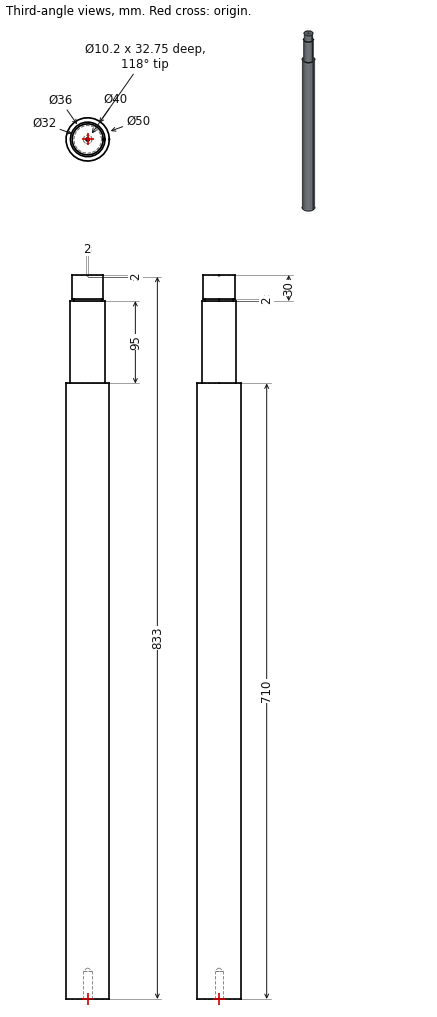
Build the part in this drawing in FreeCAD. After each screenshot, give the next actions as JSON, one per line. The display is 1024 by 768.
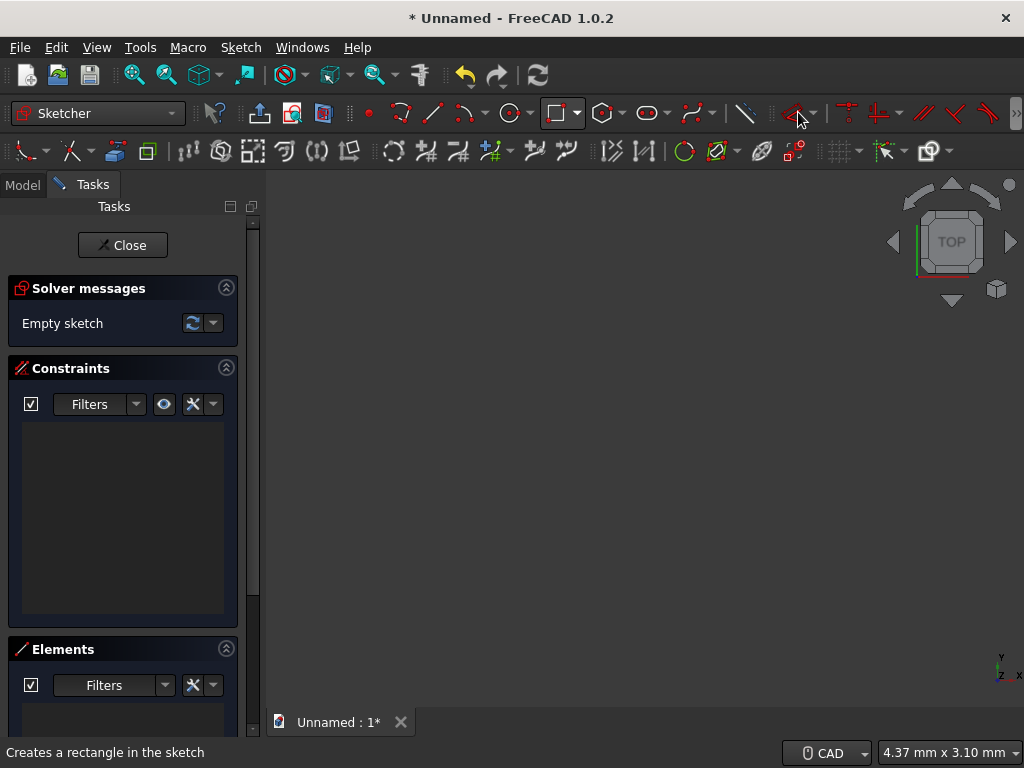
{"action": "scroll", "coordinate": [576, 438], "scroll_direction": "down", "scroll_amount": 15}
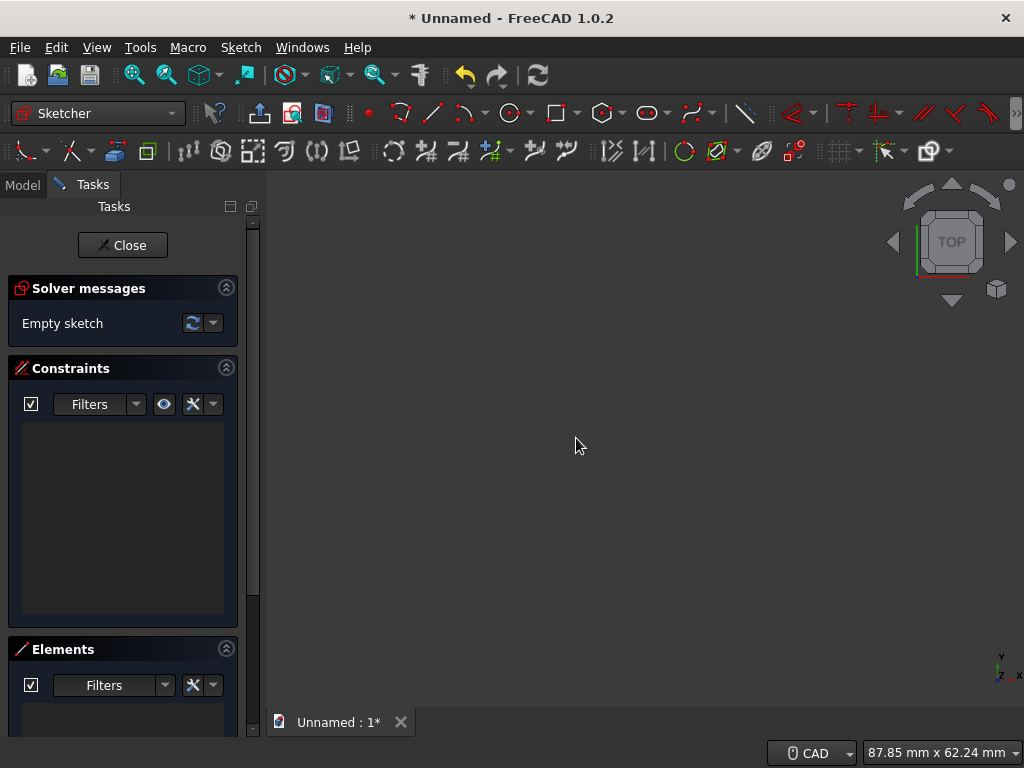
{"action": "scroll", "coordinate": [576, 438], "scroll_direction": "down", "scroll_amount": 5}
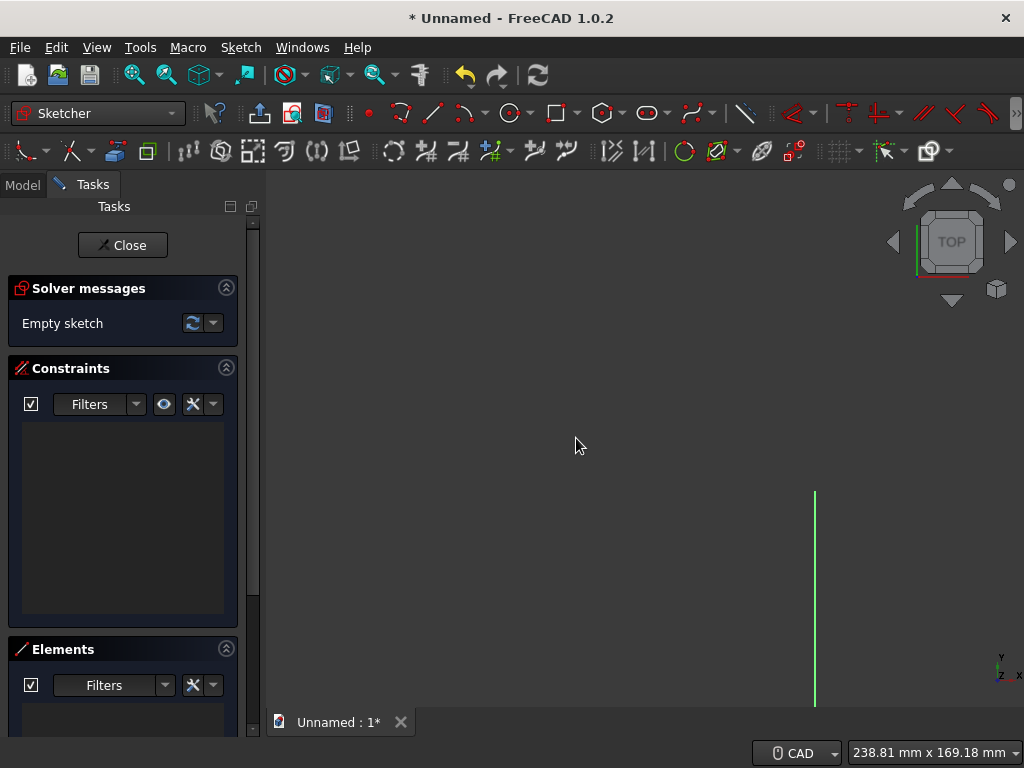
{"action": "scroll", "coordinate": [576, 438], "scroll_direction": "down", "scroll_amount": 5}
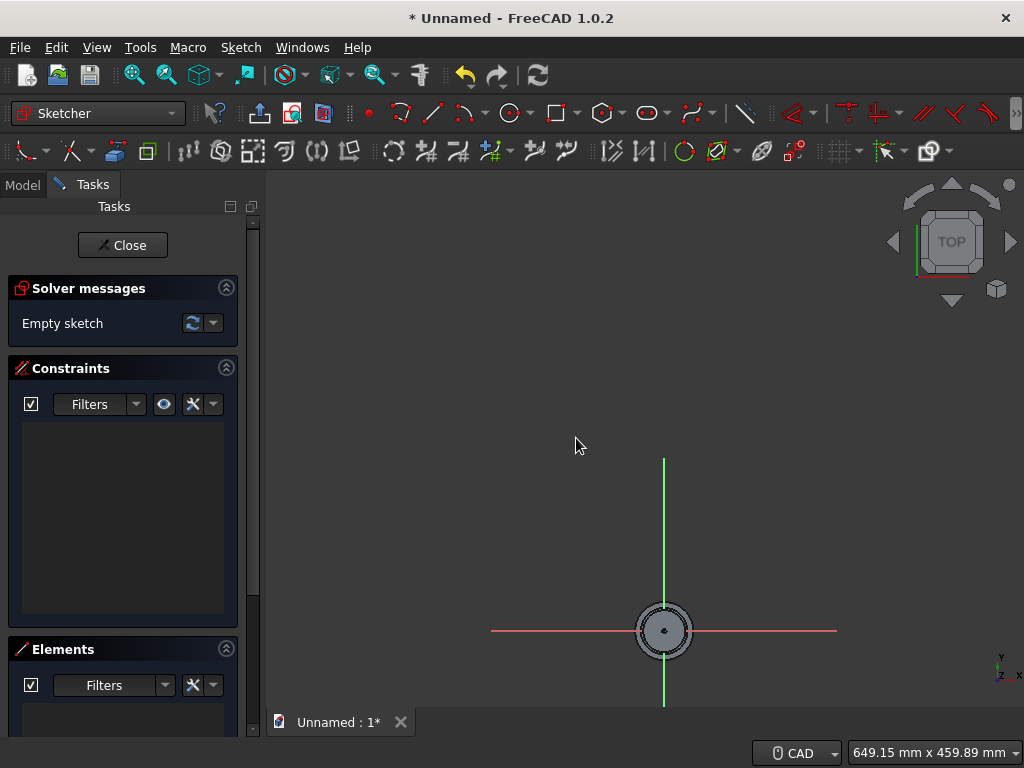
{"action": "scroll", "coordinate": [678, 661], "scroll_direction": "up", "scroll_amount": 10}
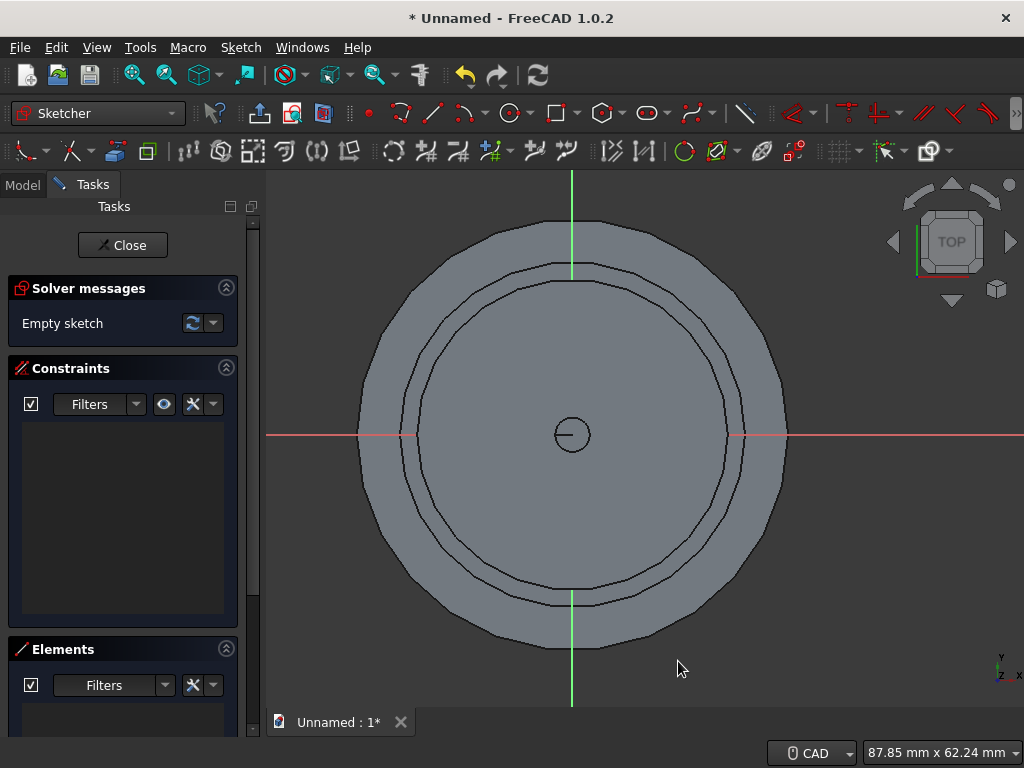
{"action": "left_click", "coordinate": [510, 114]}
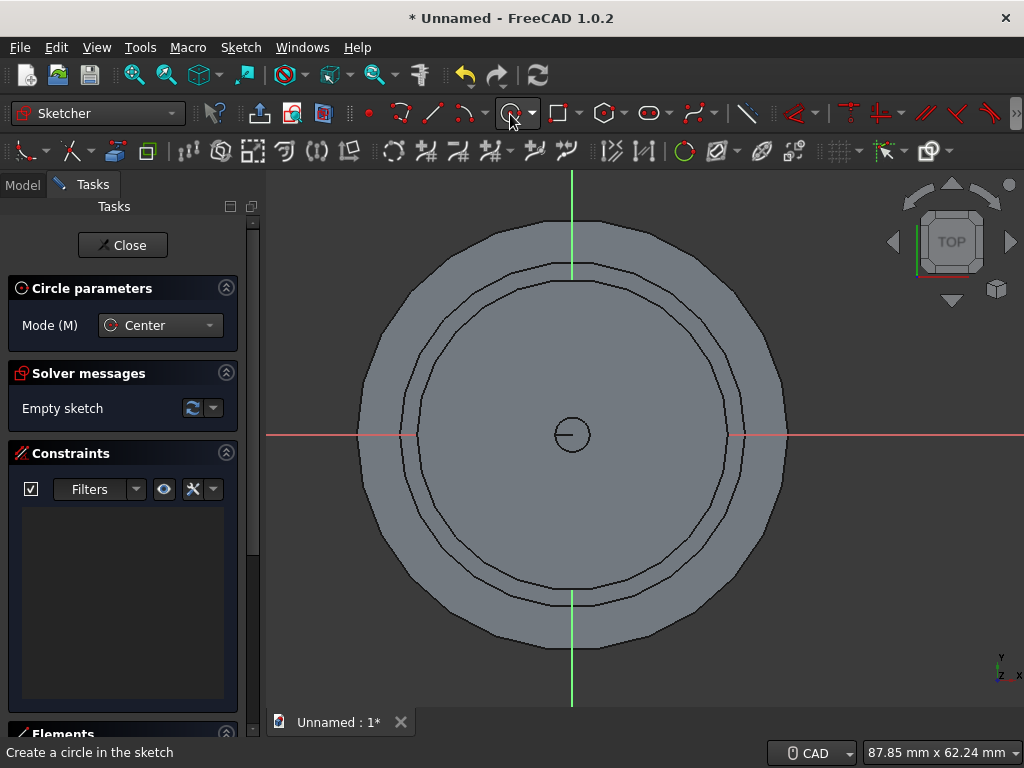
{"action": "left_click", "coordinate": [572, 435]}
{"action": "mouse_move", "coordinate": [695, 313]}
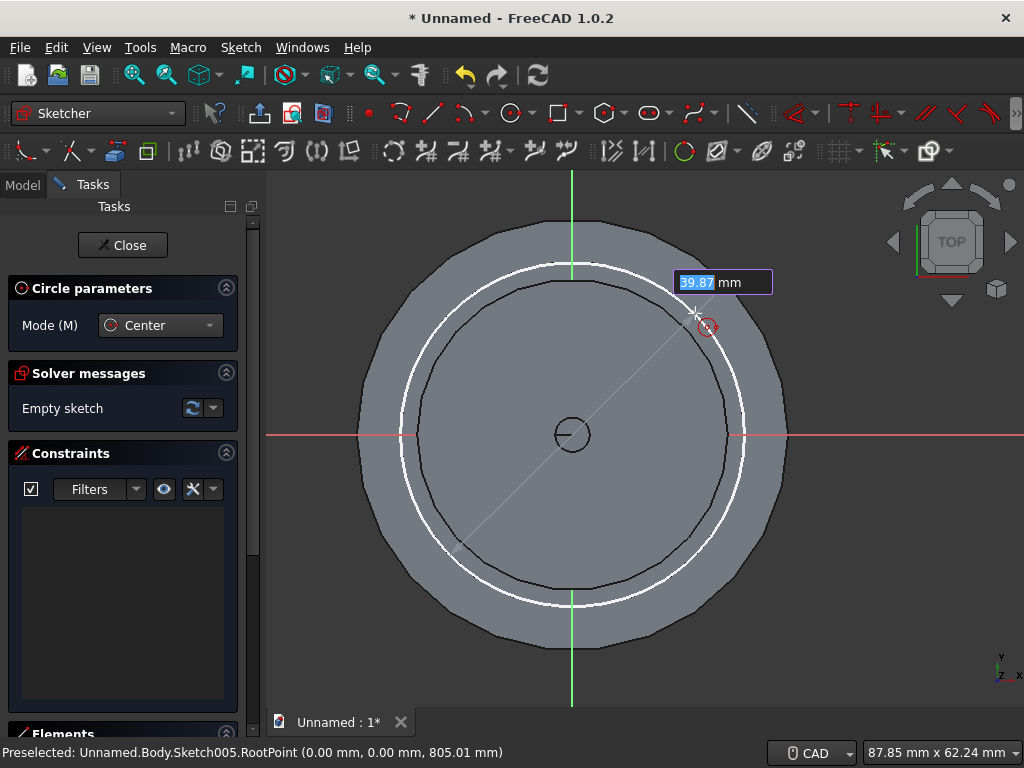
{"action": "type", "text": "40"}
{"action": "key", "text": "Return"}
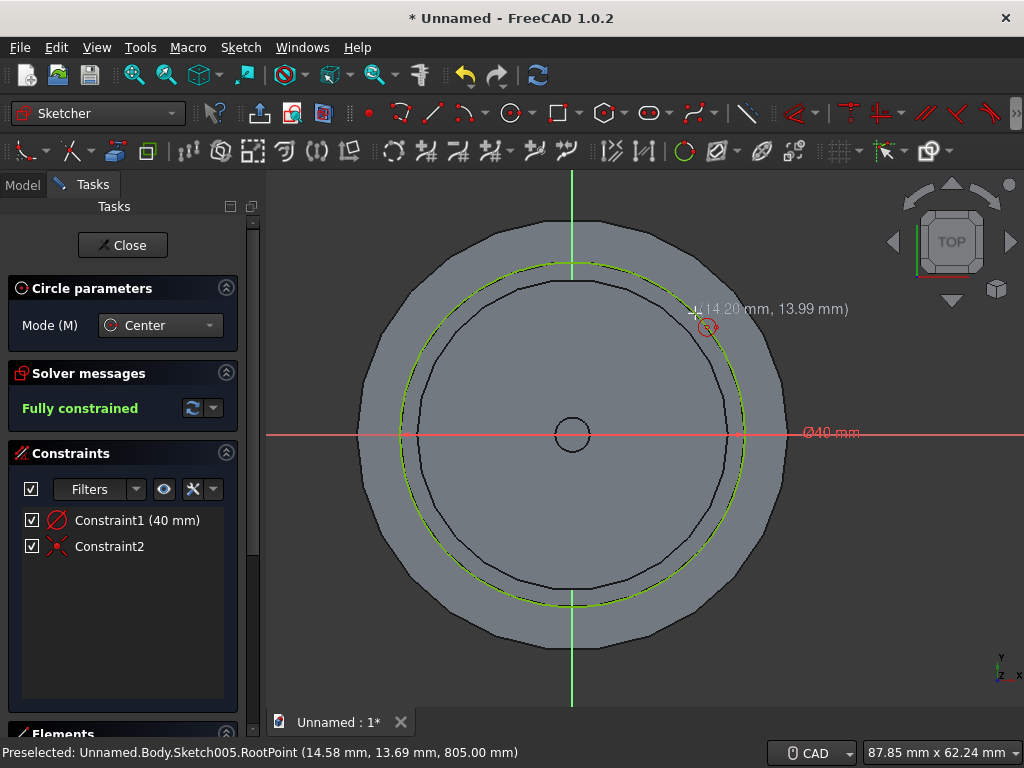
{"action": "left_click", "coordinate": [572, 435]}
{"action": "mouse_move", "coordinate": [670, 337]}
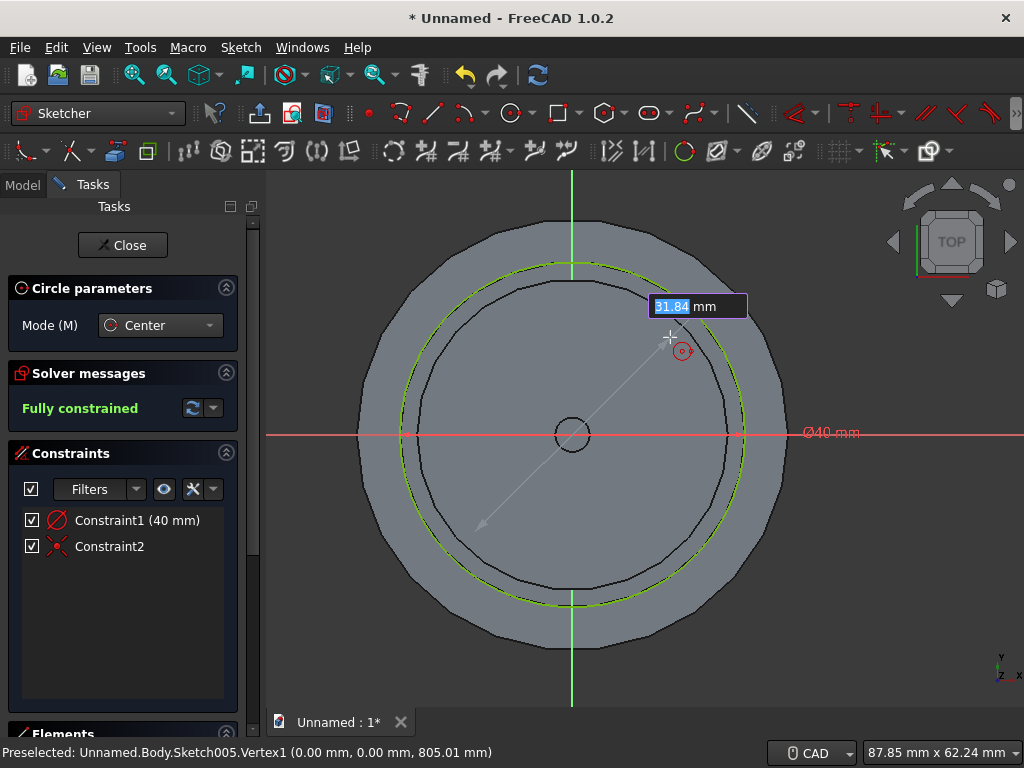
{"action": "type", "text": "32"}
{"action": "key", "text": "Return"}
{"action": "key", "text": "Escape"}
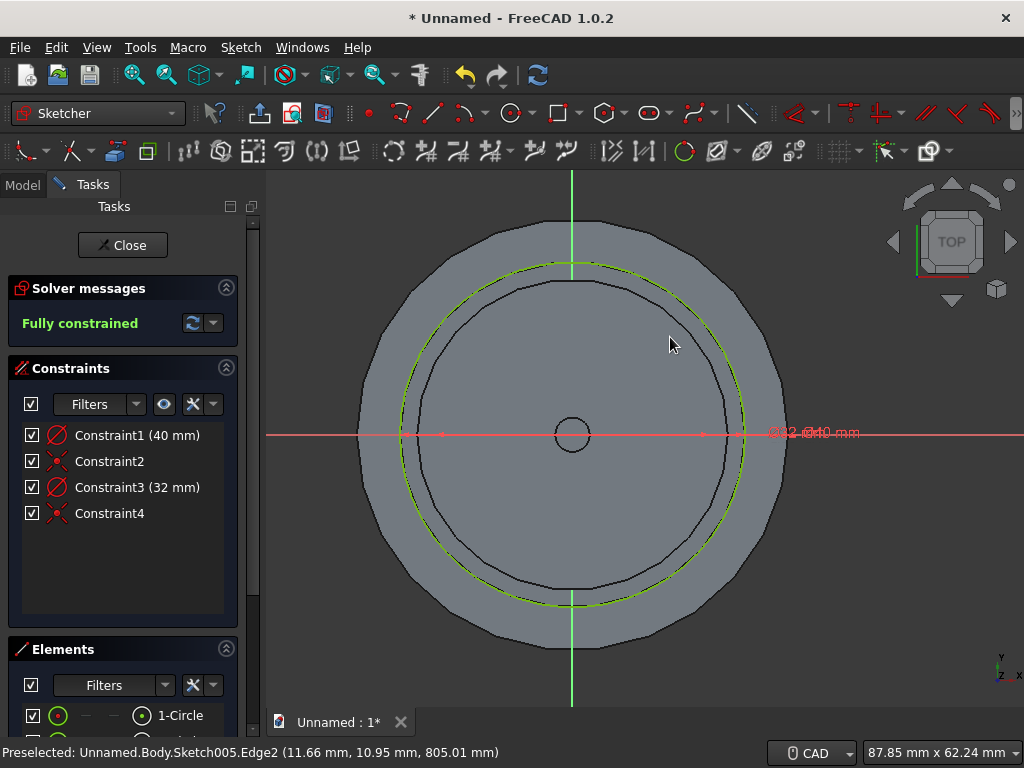
{"action": "left_click", "coordinate": [123, 245]}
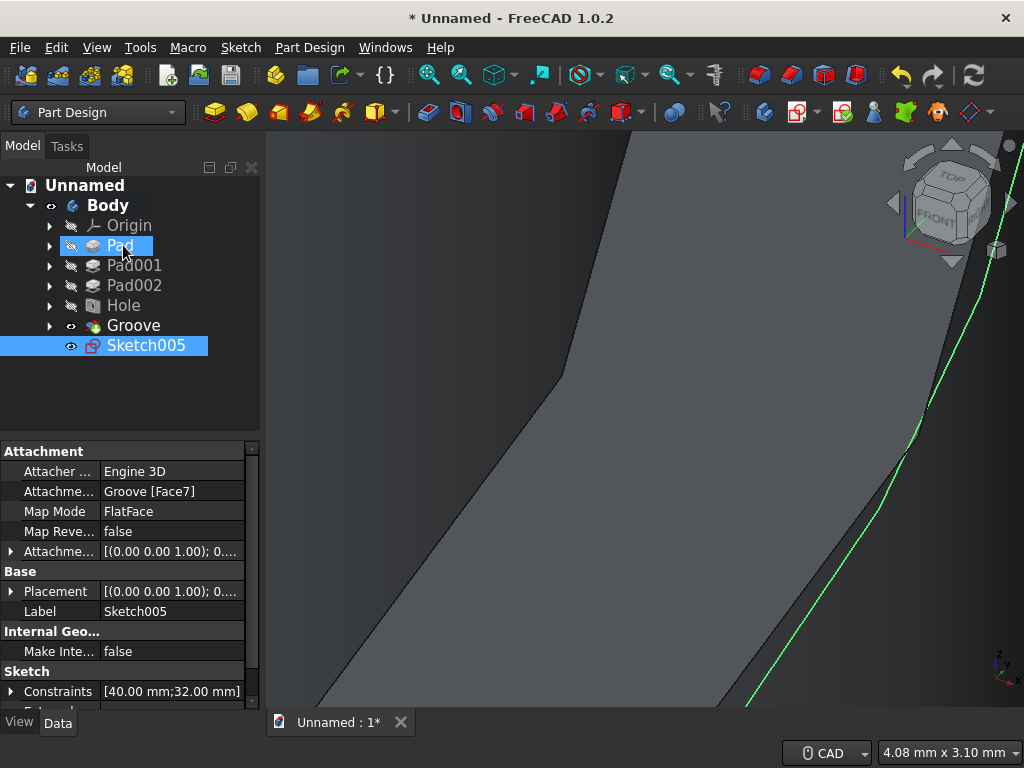
{"action": "left_click", "coordinate": [430, 112]}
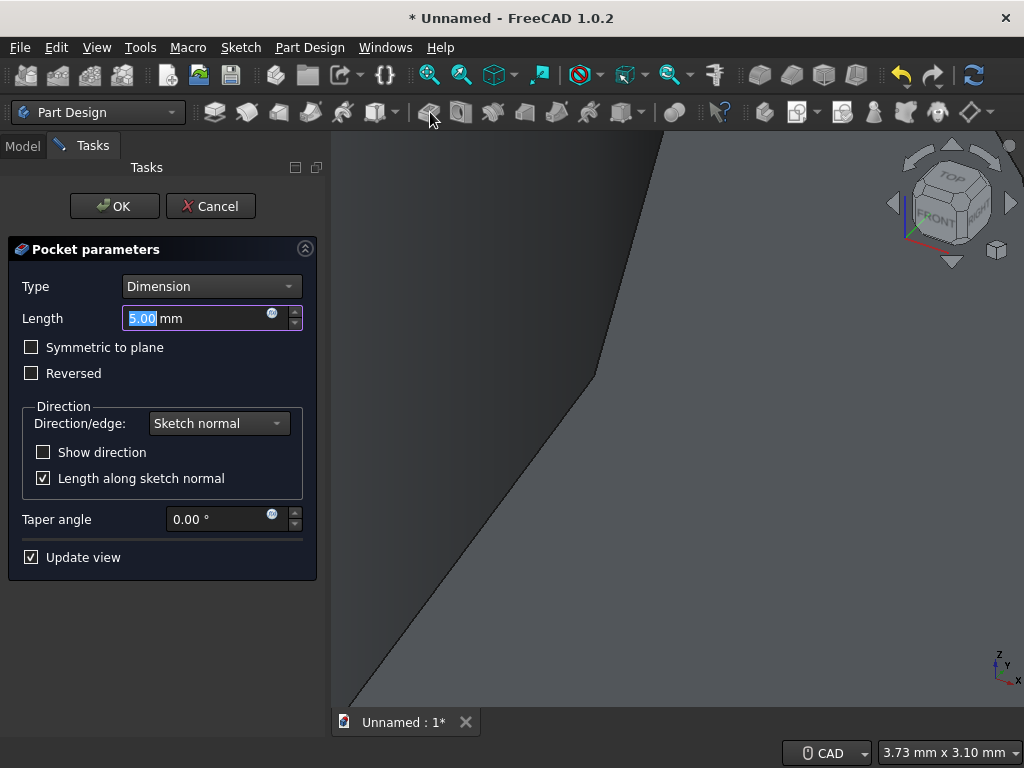
{"action": "type", "text": "2"}
{"action": "key", "text": "Tab"}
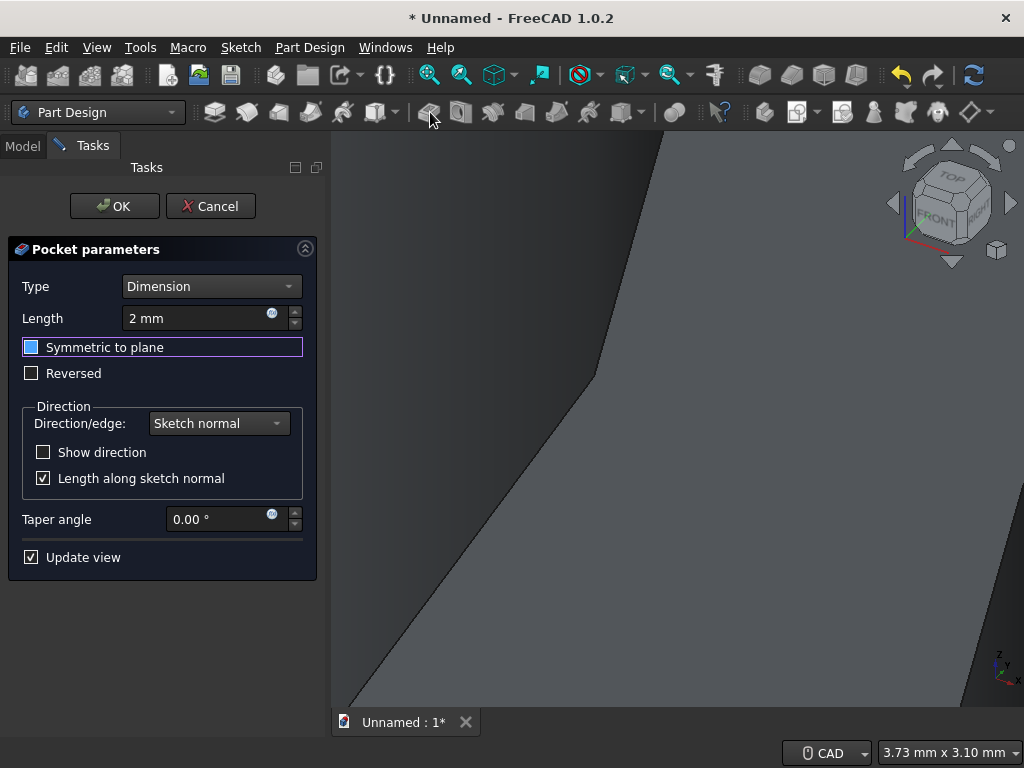
{"action": "left_click", "coordinate": [30, 373]}